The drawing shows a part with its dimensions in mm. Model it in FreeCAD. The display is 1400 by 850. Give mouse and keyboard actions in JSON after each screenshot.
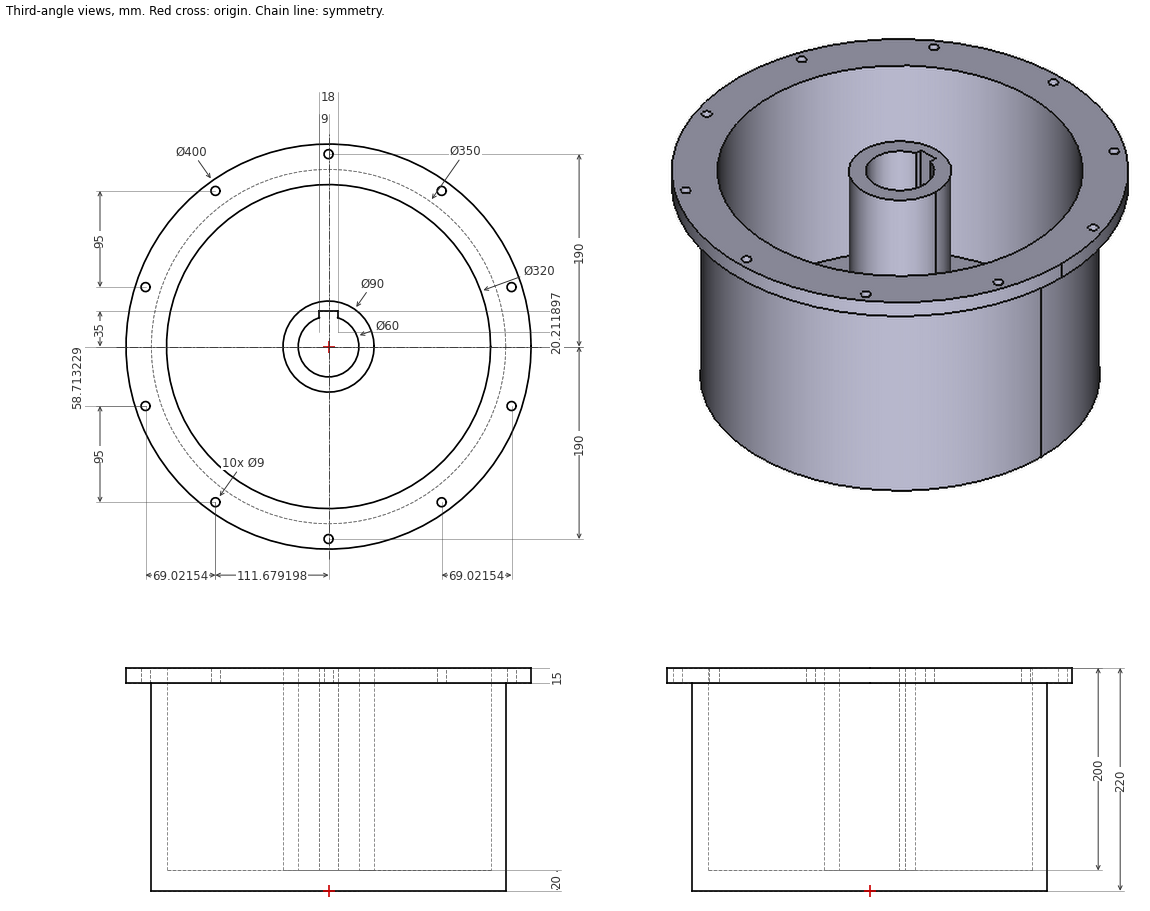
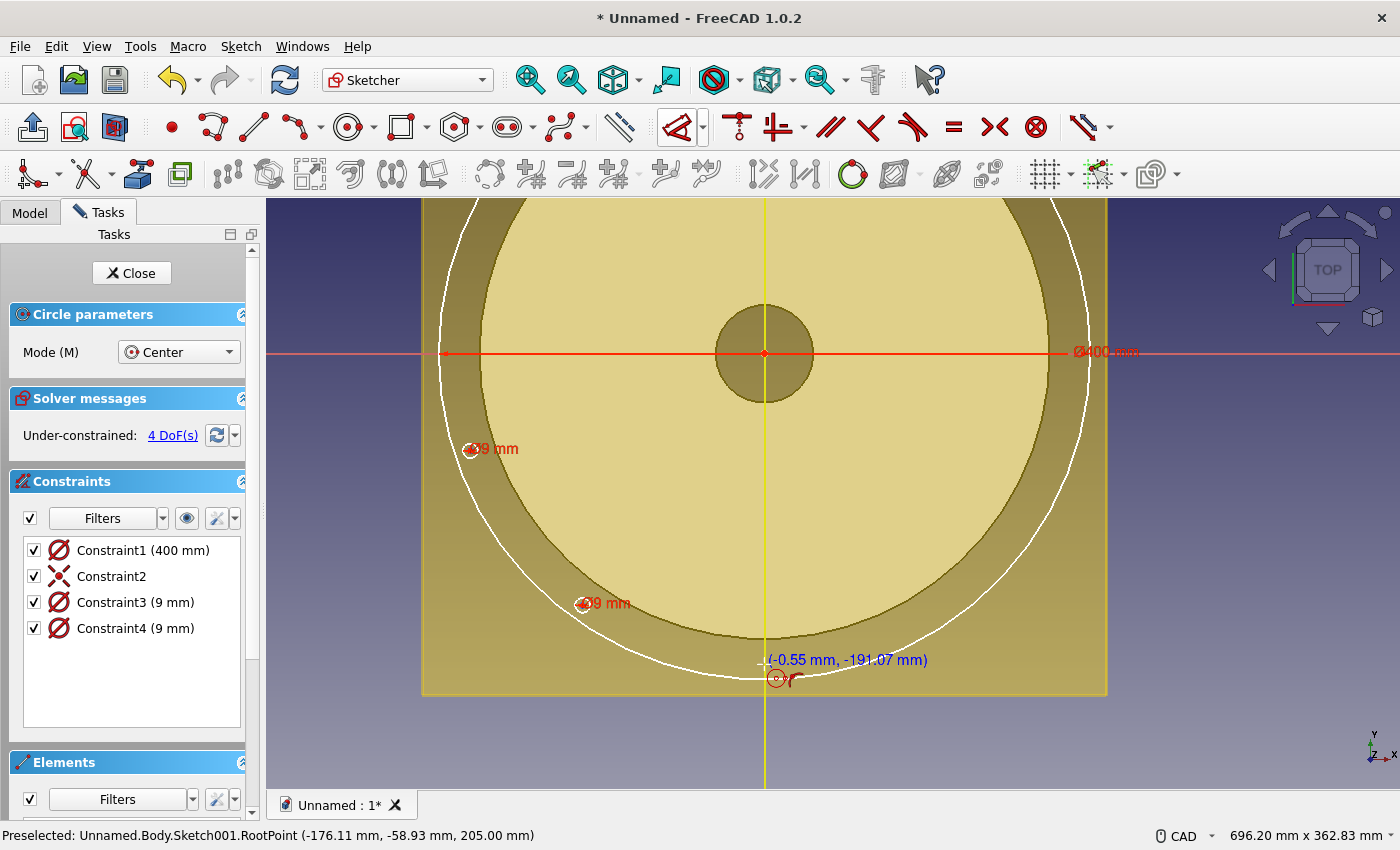
{"action": "left_click", "coordinate": [765, 663]}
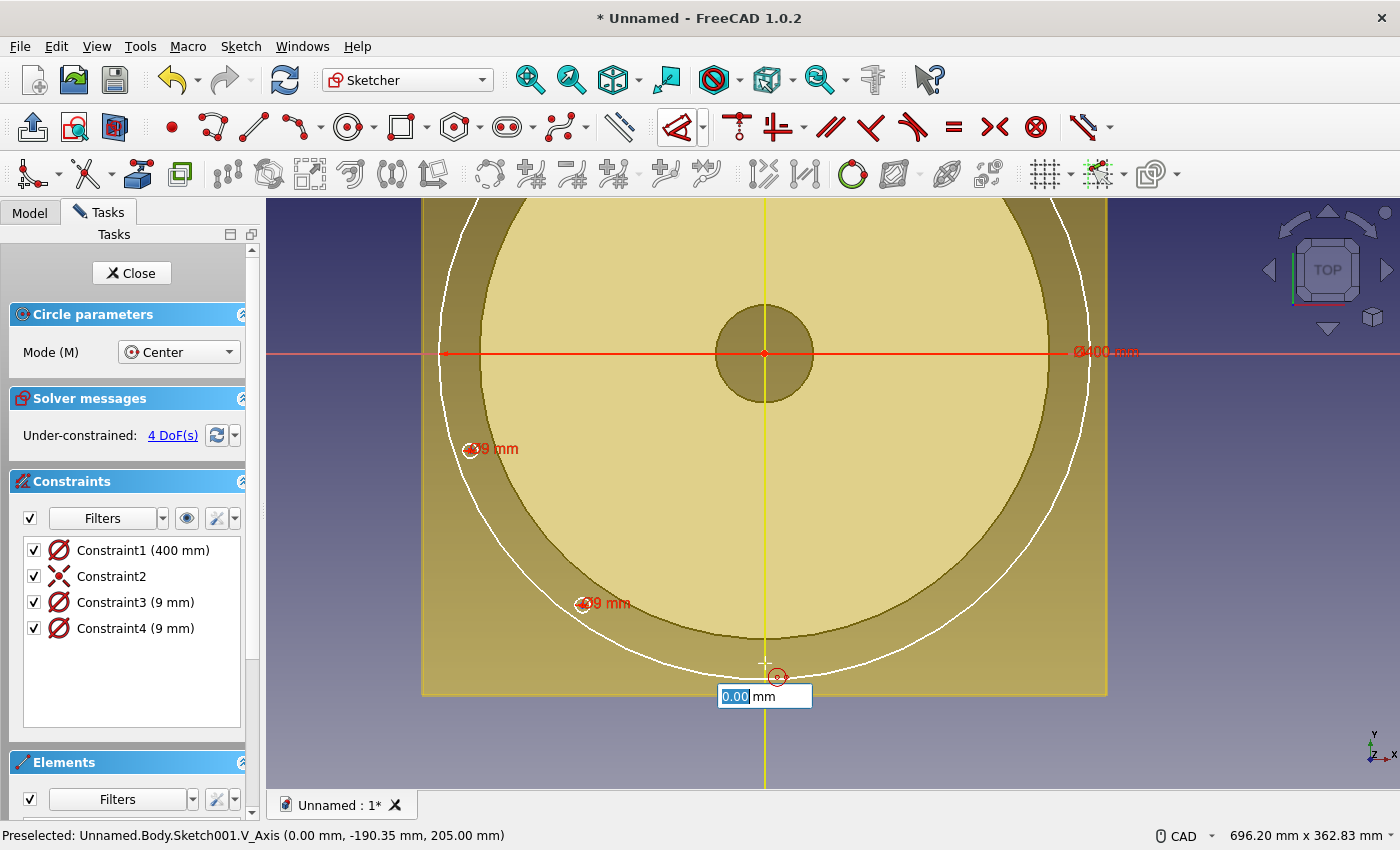
{"action": "scroll", "coordinate": [771, 661], "scroll_direction": "up", "scroll_amount": 5}
{"action": "mouse_move", "coordinate": [771, 659]}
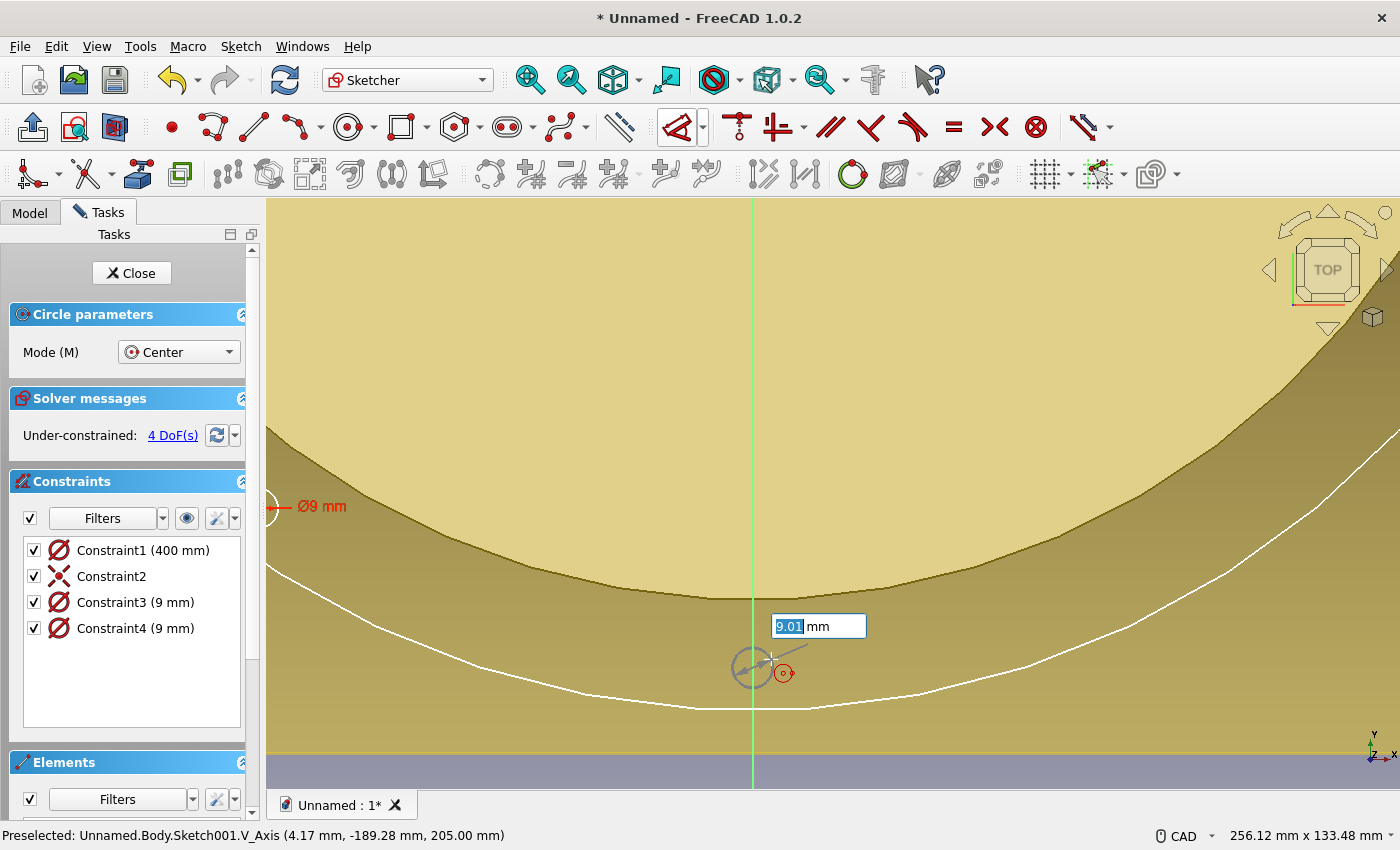
{"action": "type", "text": "9"}
{"action": "key", "text": "Return"}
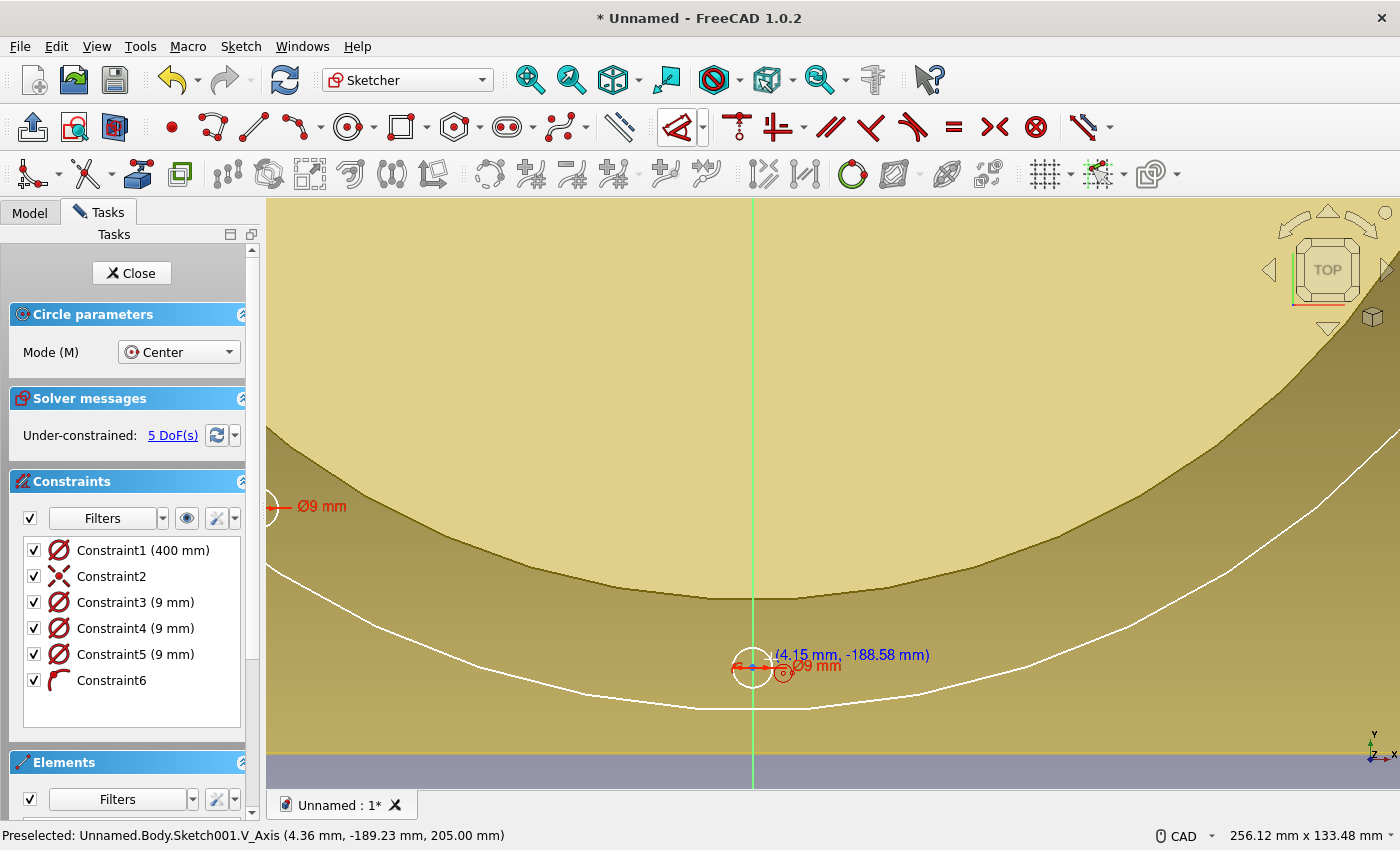
{"action": "scroll", "coordinate": [768, 663], "scroll_direction": "down", "scroll_amount": 8}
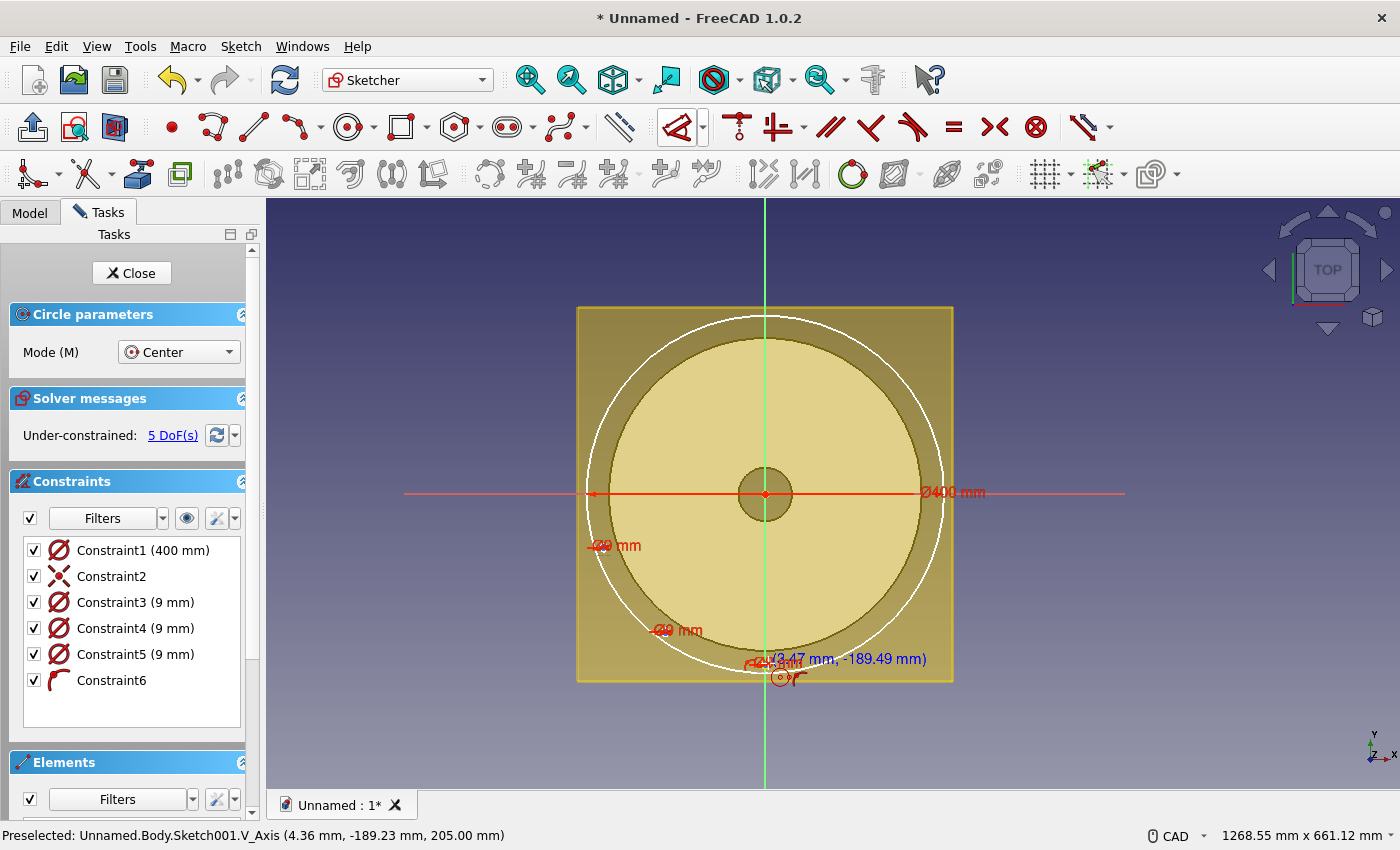
{"action": "scroll", "coordinate": [865, 632], "scroll_direction": "up", "scroll_amount": 9}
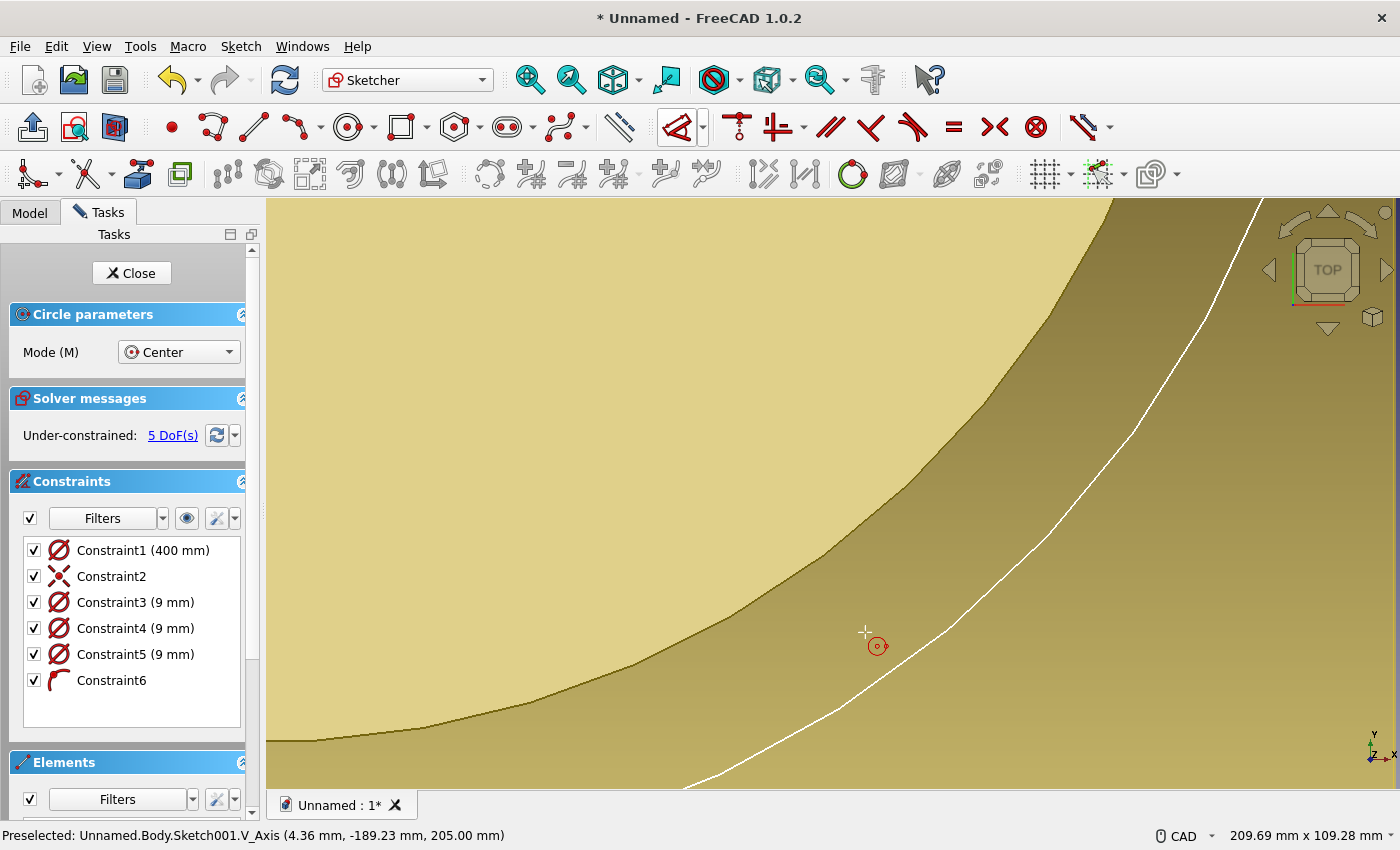
{"action": "scroll", "coordinate": [865, 632], "scroll_direction": "down", "scroll_amount": 9}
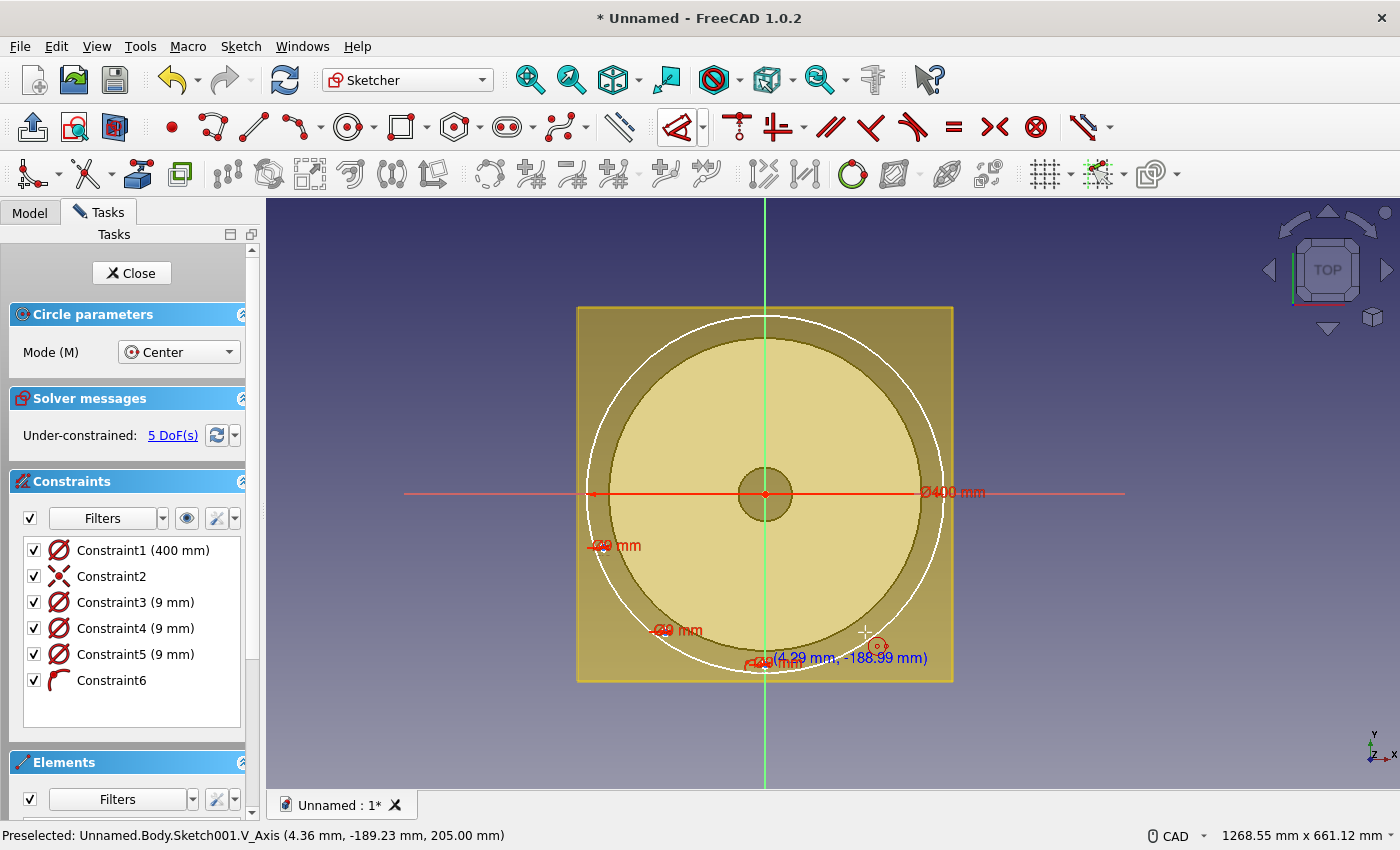
{"action": "scroll", "coordinate": [865, 632], "scroll_direction": "up", "scroll_amount": 3}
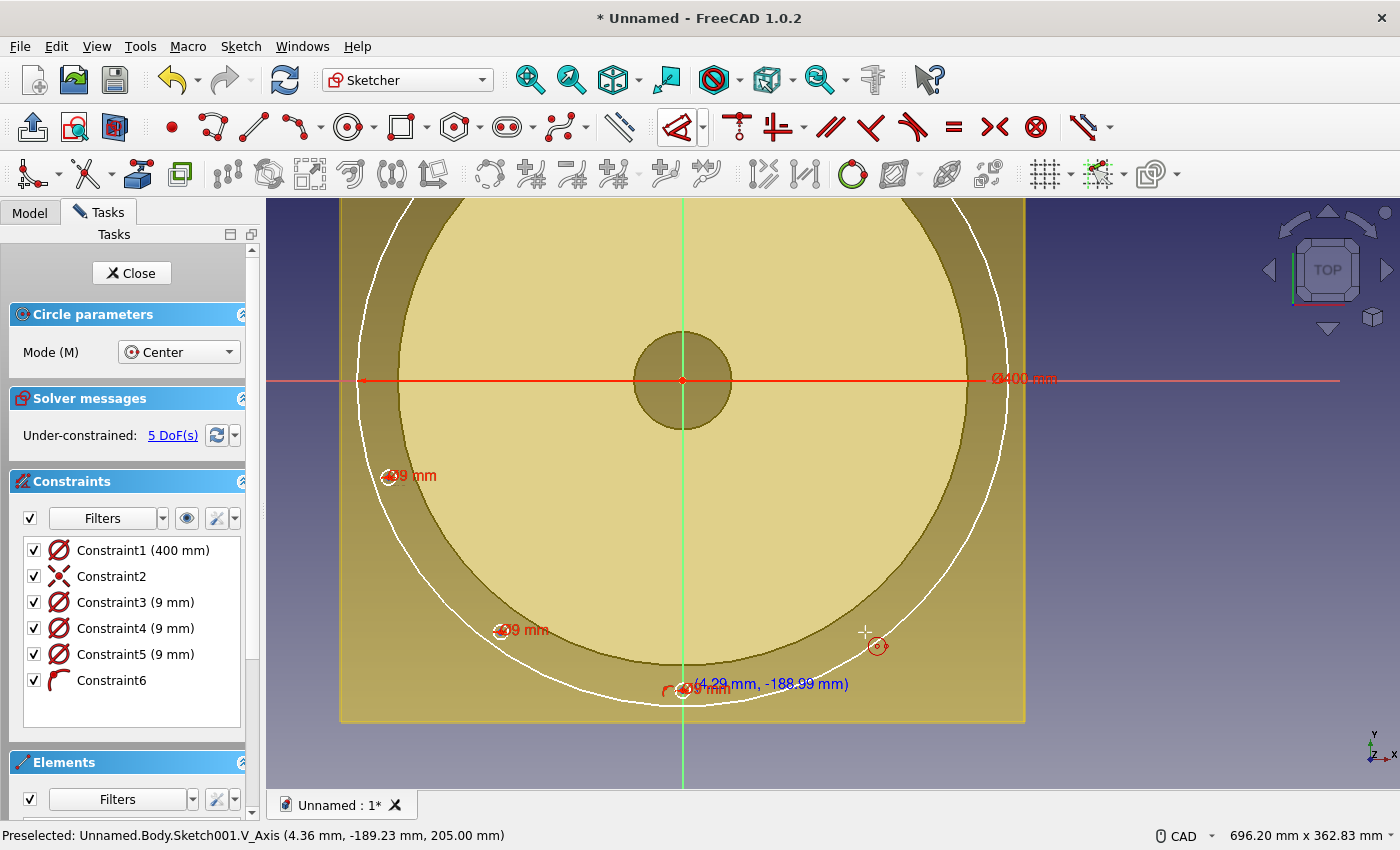
{"action": "left_click", "coordinate": [865, 631]}
{"action": "mouse_move", "coordinate": [870, 626]}